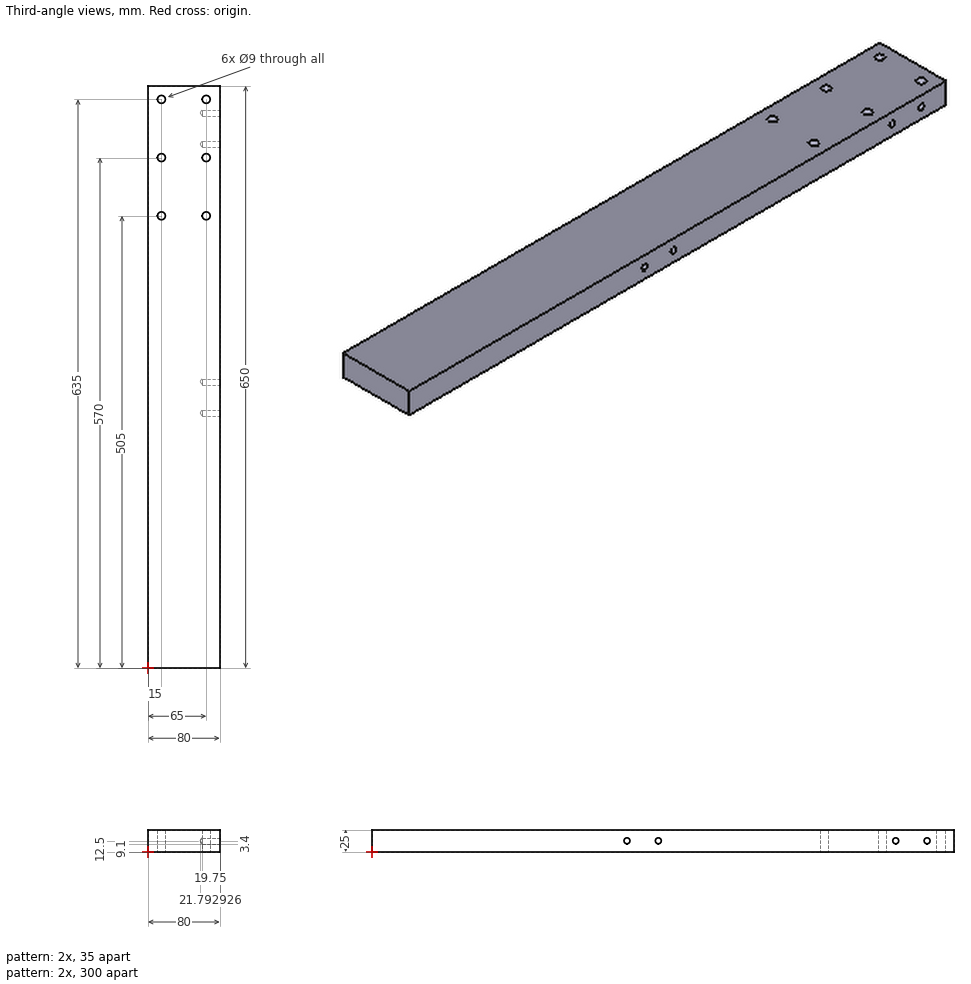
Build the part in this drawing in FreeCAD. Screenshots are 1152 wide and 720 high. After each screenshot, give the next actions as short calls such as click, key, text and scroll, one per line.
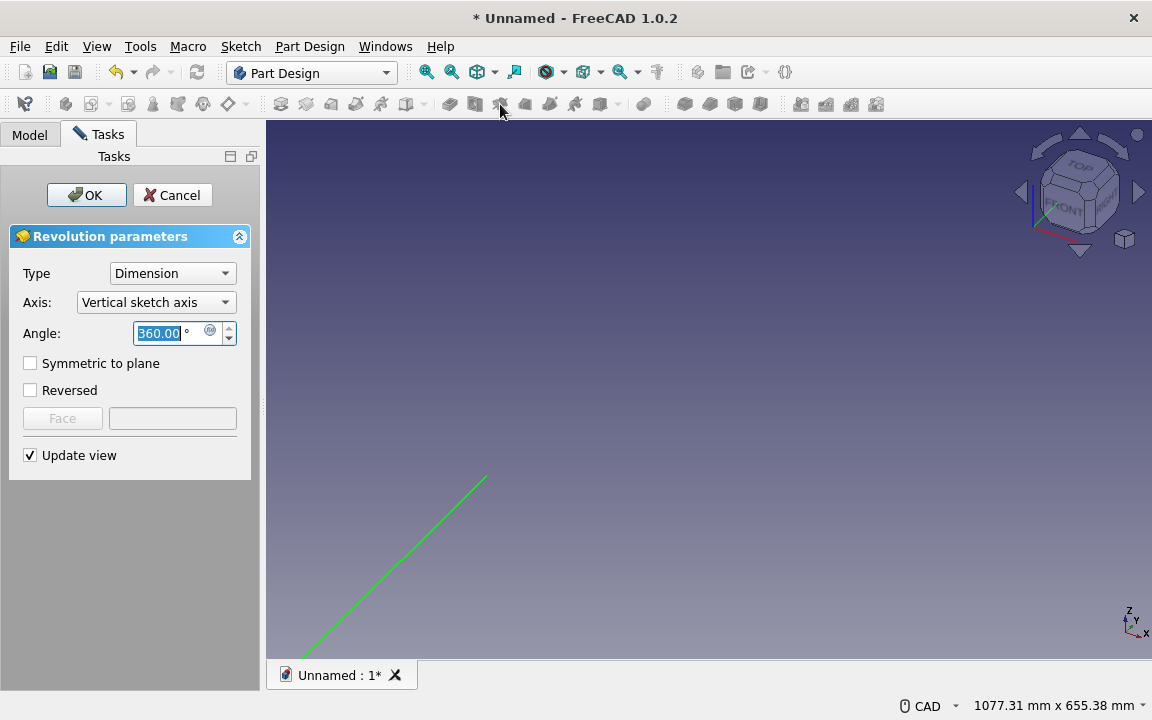
click(157, 302)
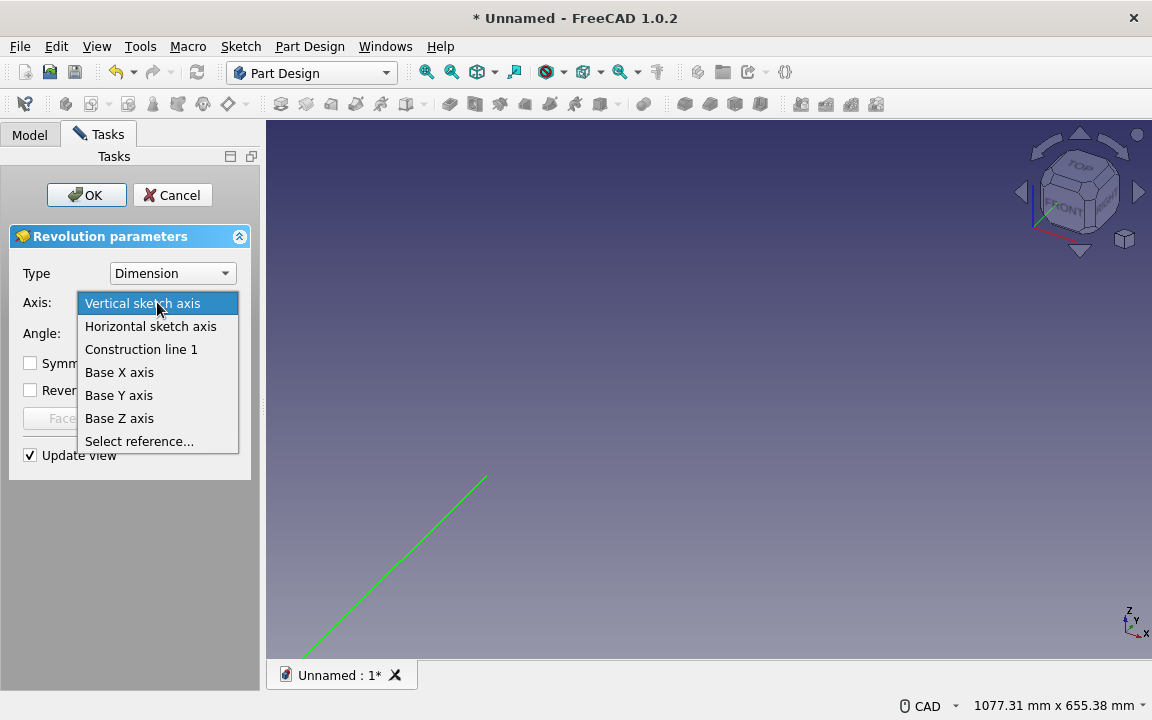
click(156, 350)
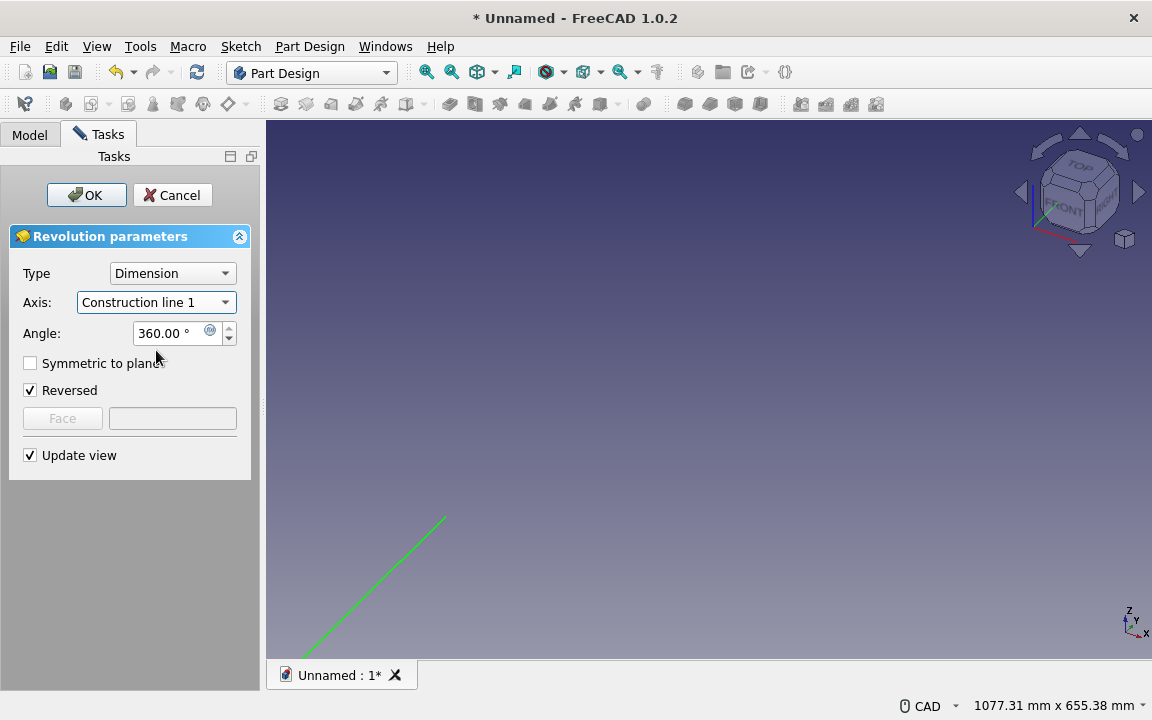
click(87, 195)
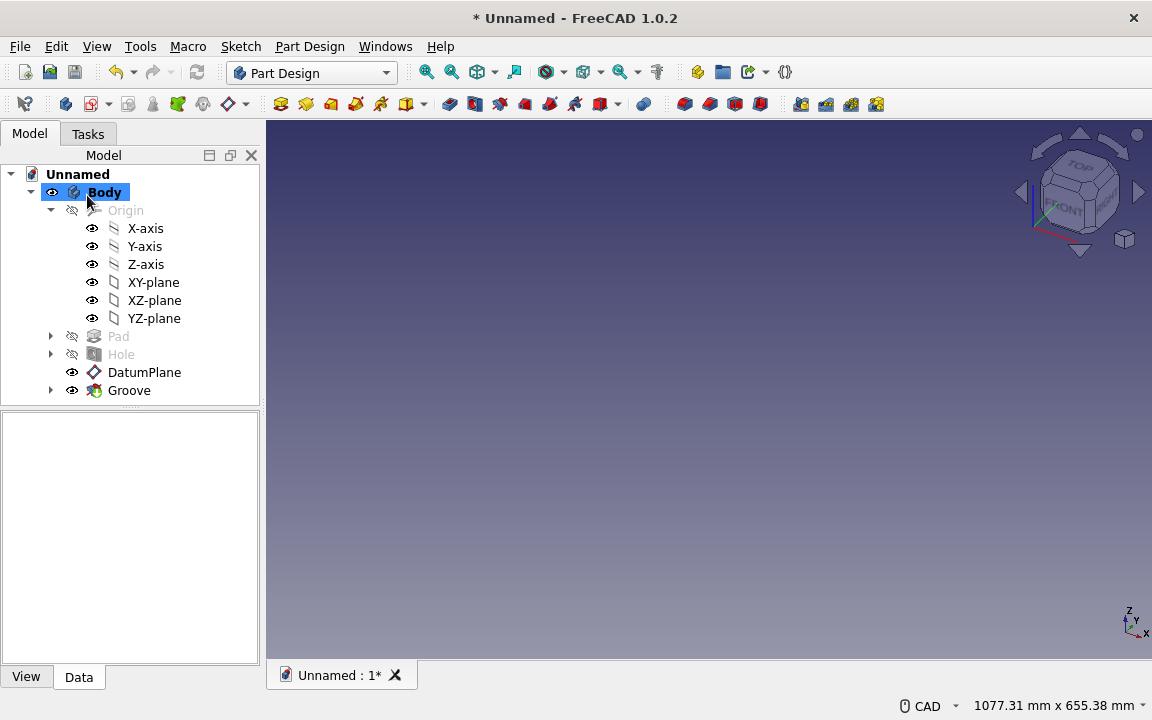
click(117, 372)
key(space)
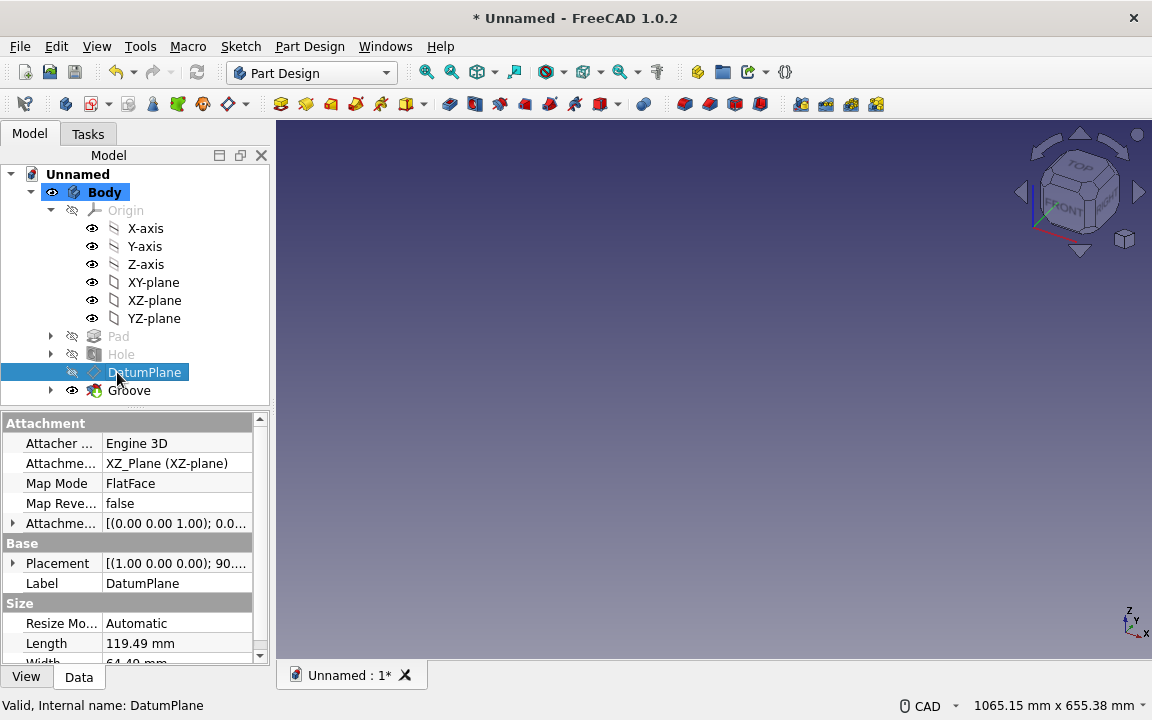
key(v)
key(f)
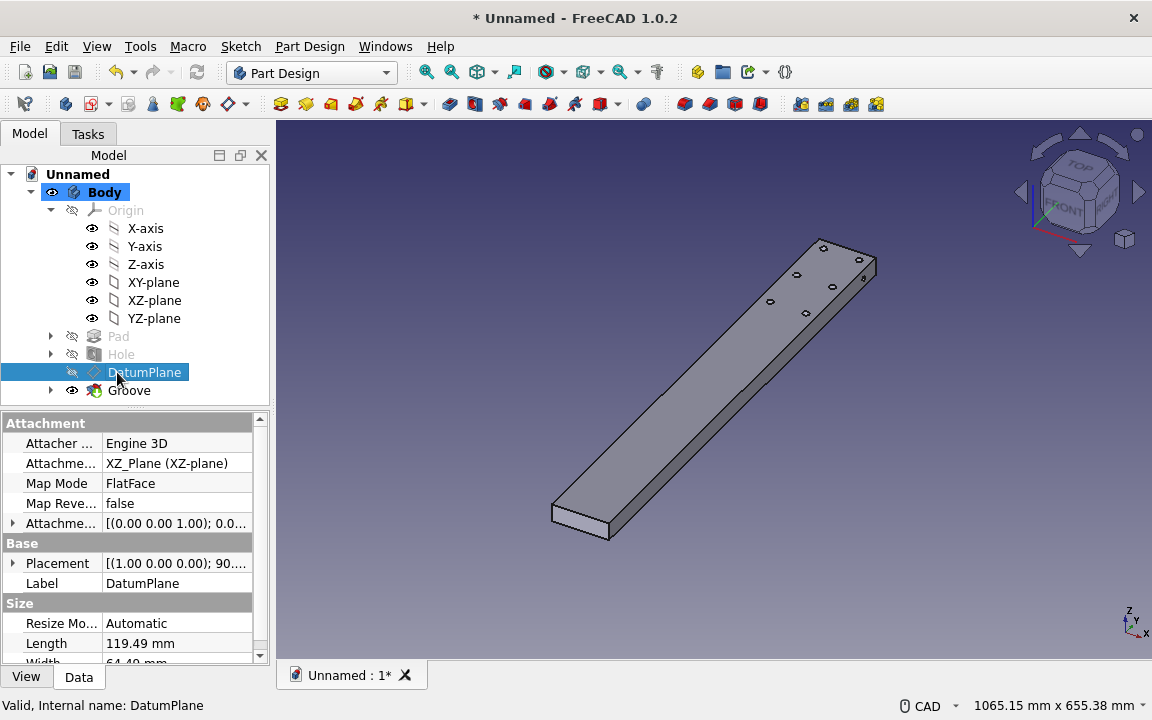
click(117, 390)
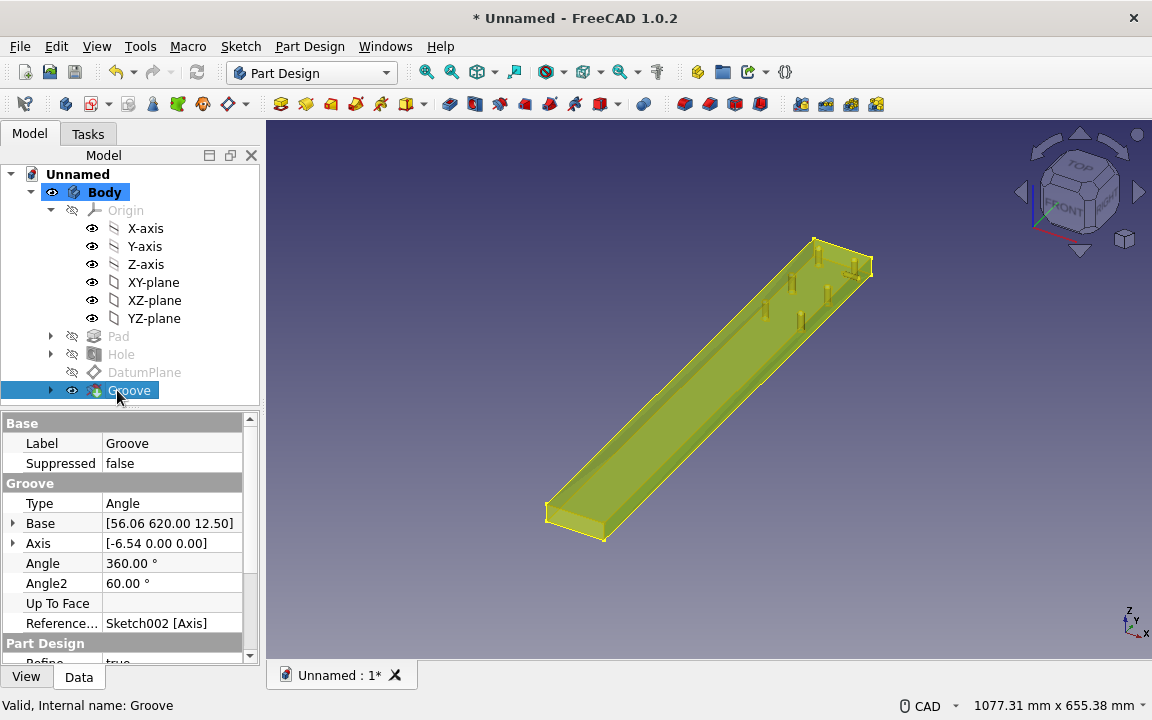
click(826, 104)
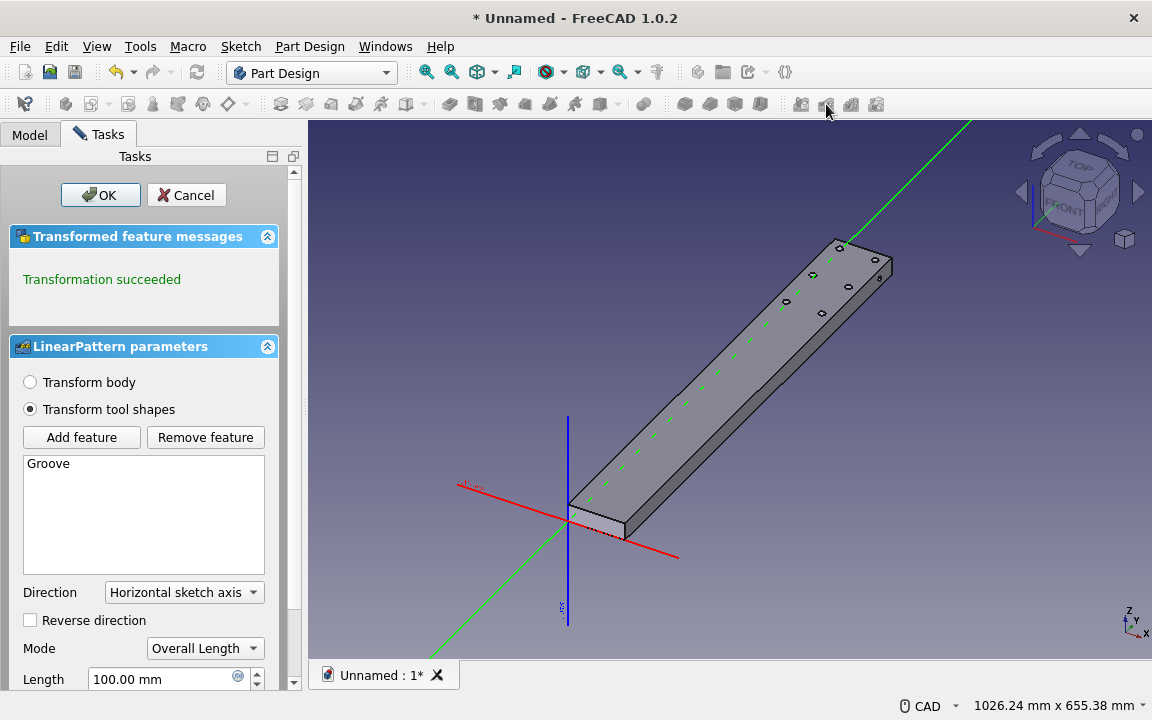
click(185, 592)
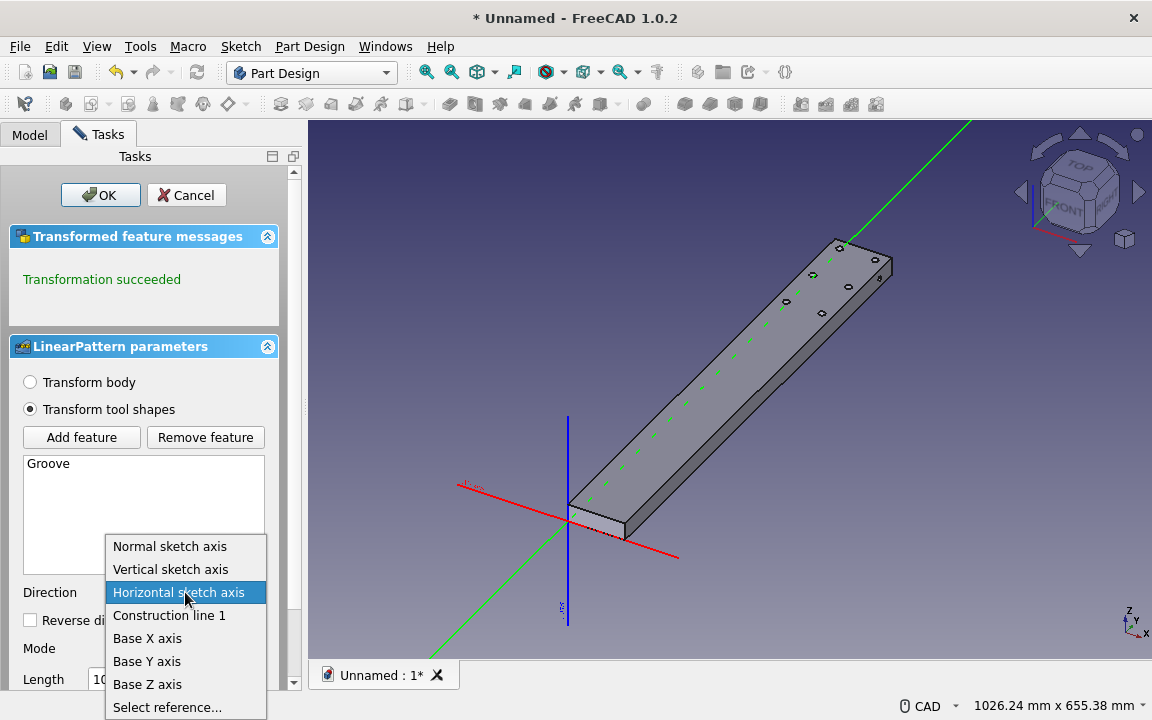
click(184, 662)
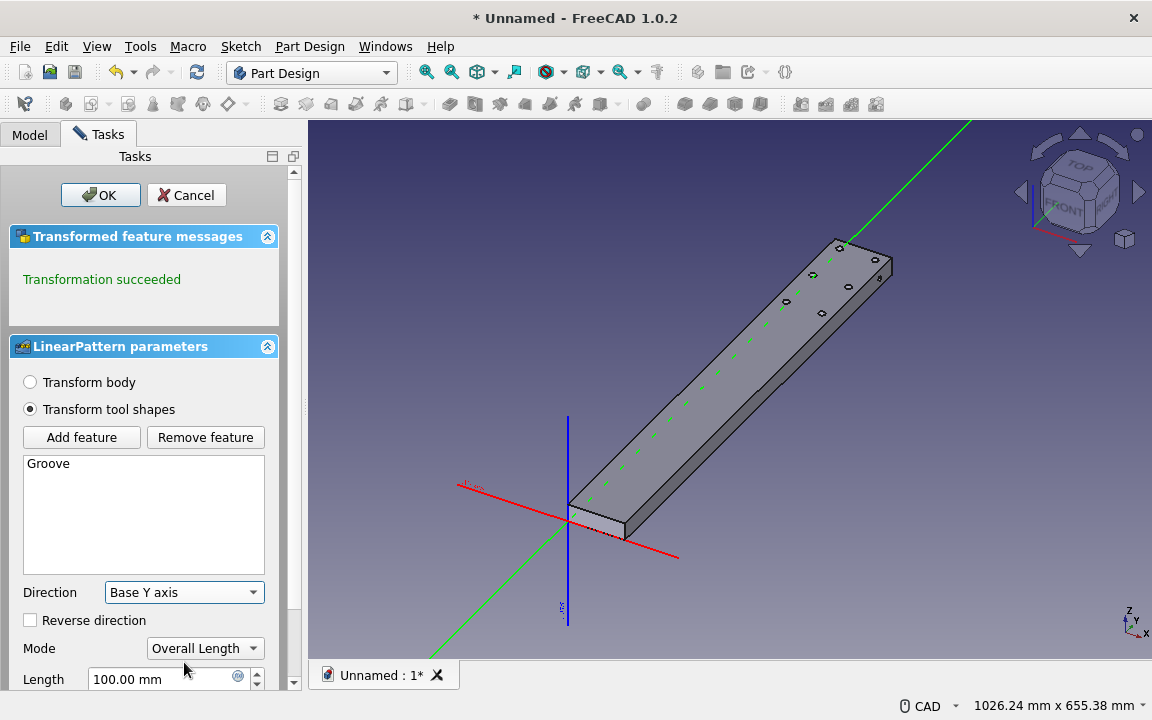
click(206, 648)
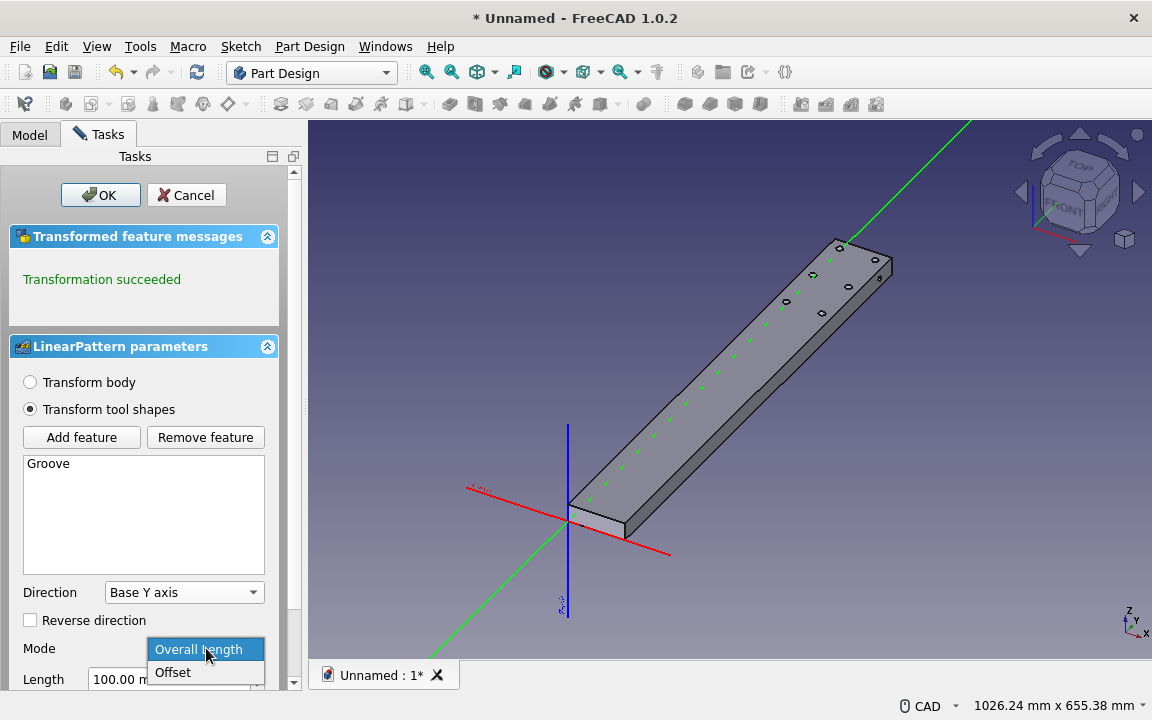
click(204, 672)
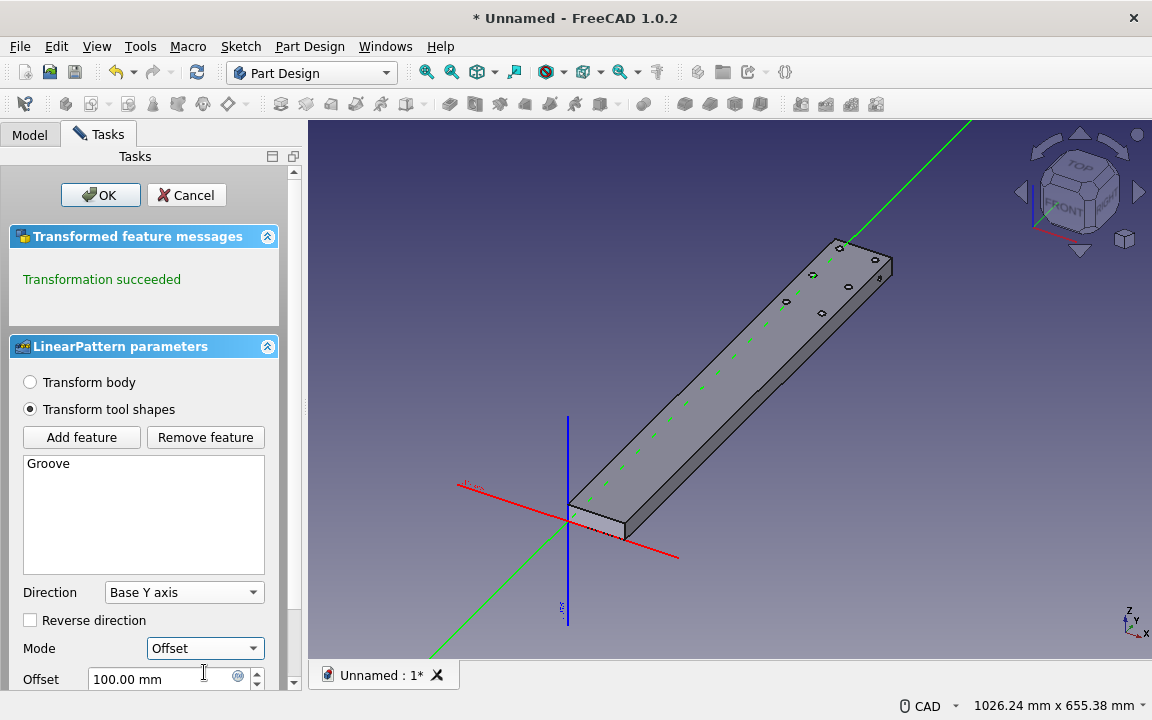
scroll(294, 428, down, 2)